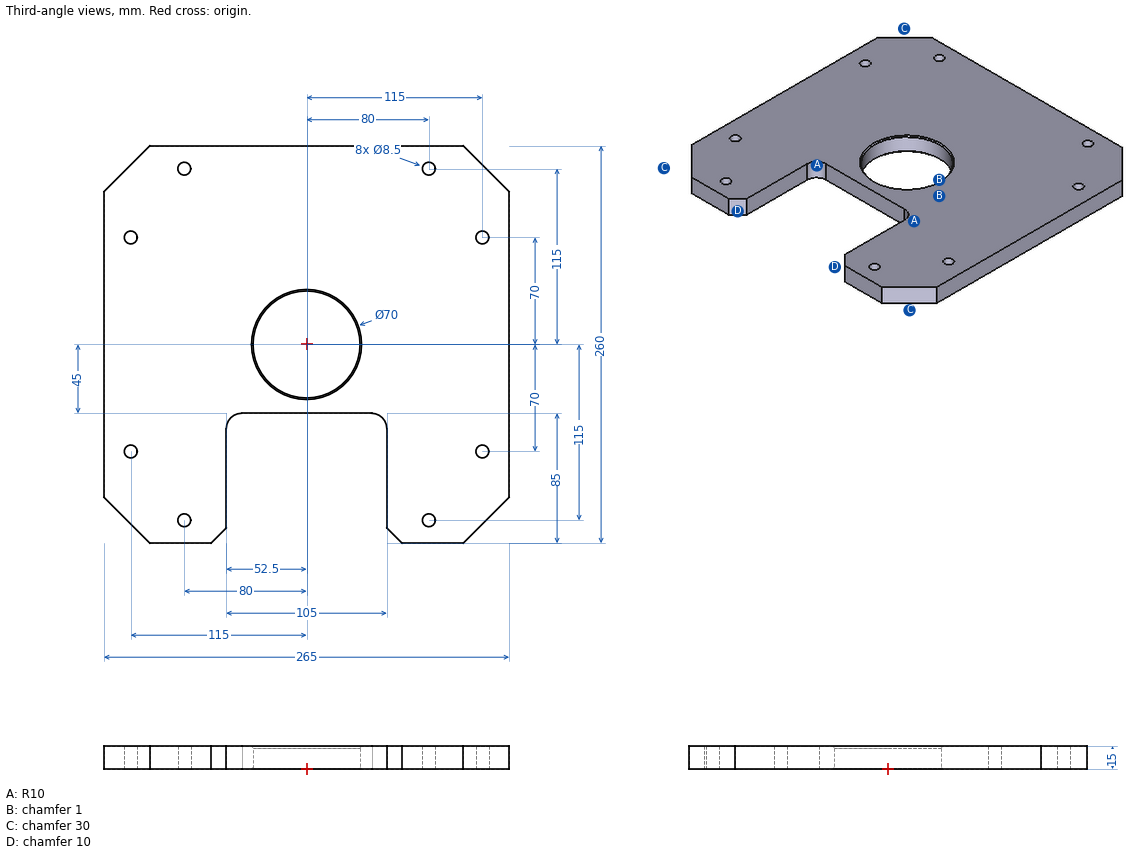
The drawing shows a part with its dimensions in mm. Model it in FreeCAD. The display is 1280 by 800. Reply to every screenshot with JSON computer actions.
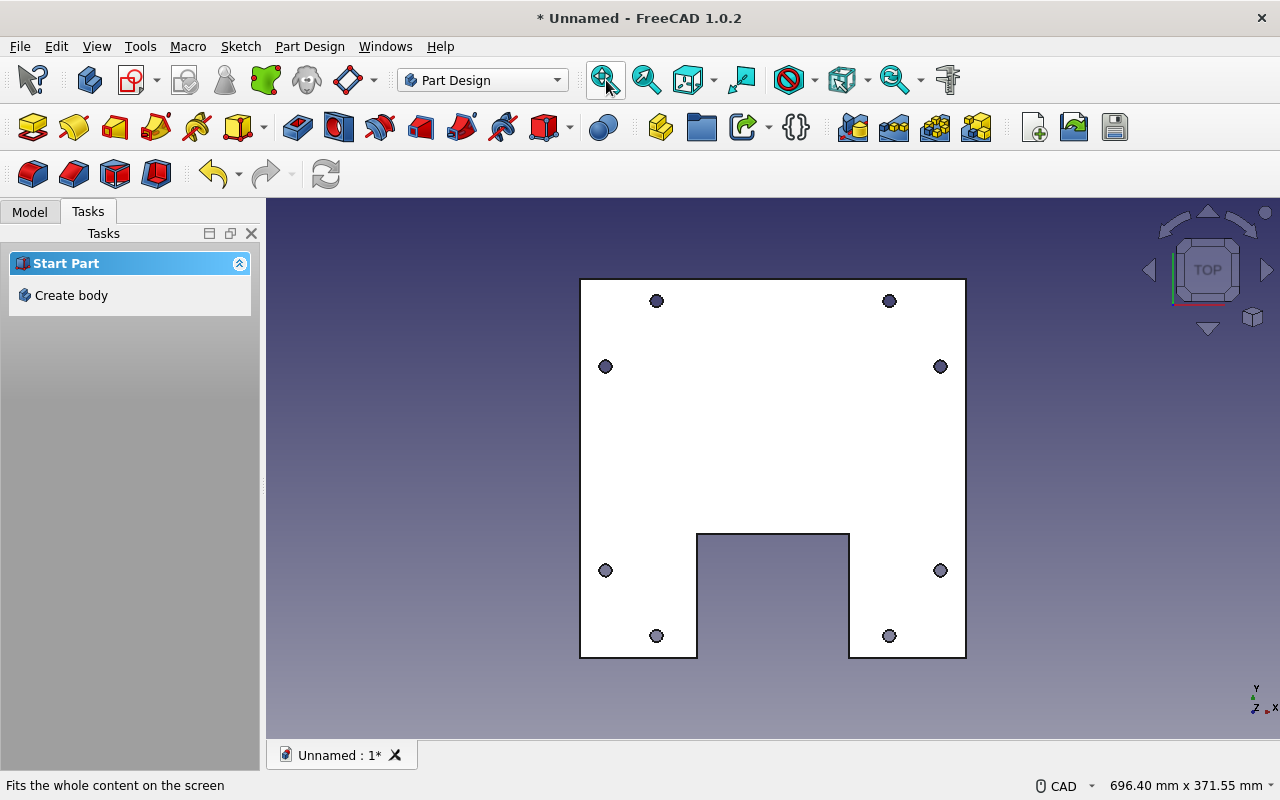
{"action": "scroll", "coordinate": [849, 533], "scroll_direction": "up", "scroll_amount": 4}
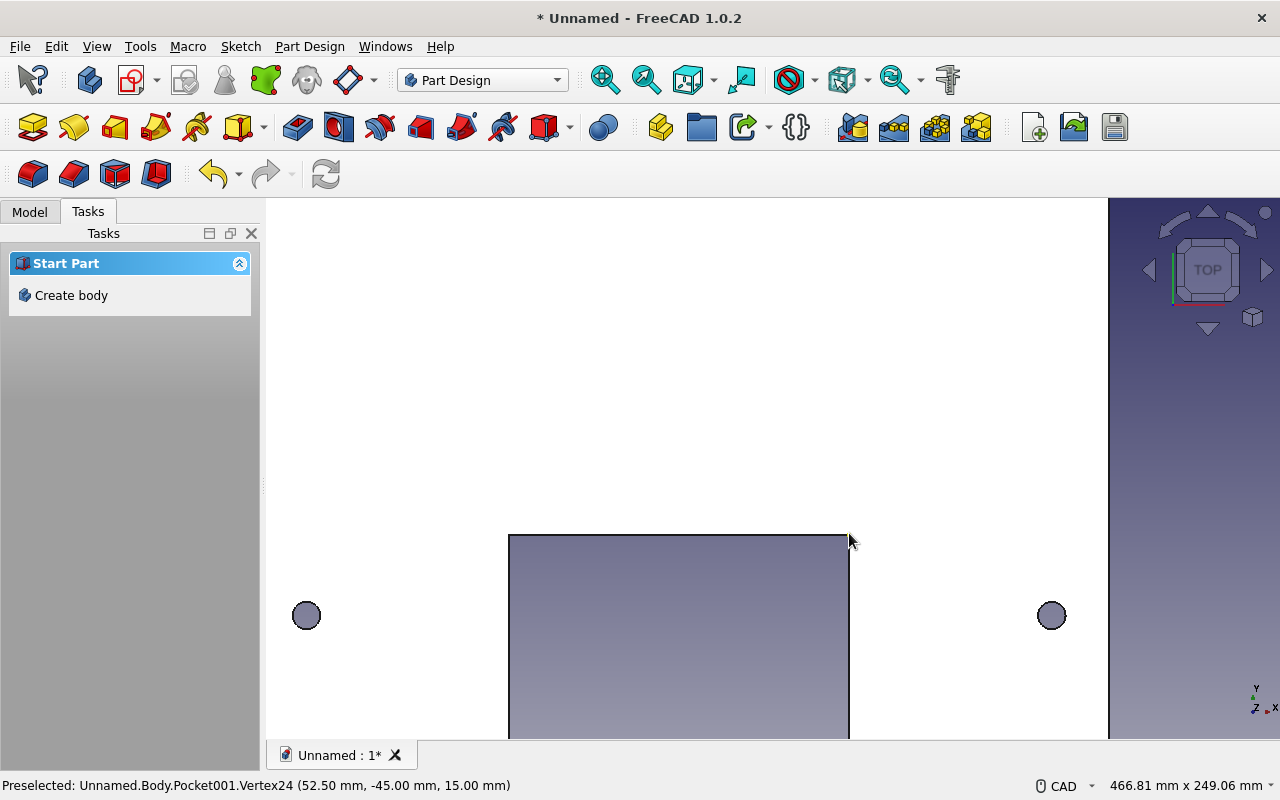
{"action": "left_click", "coordinate": [606, 80]}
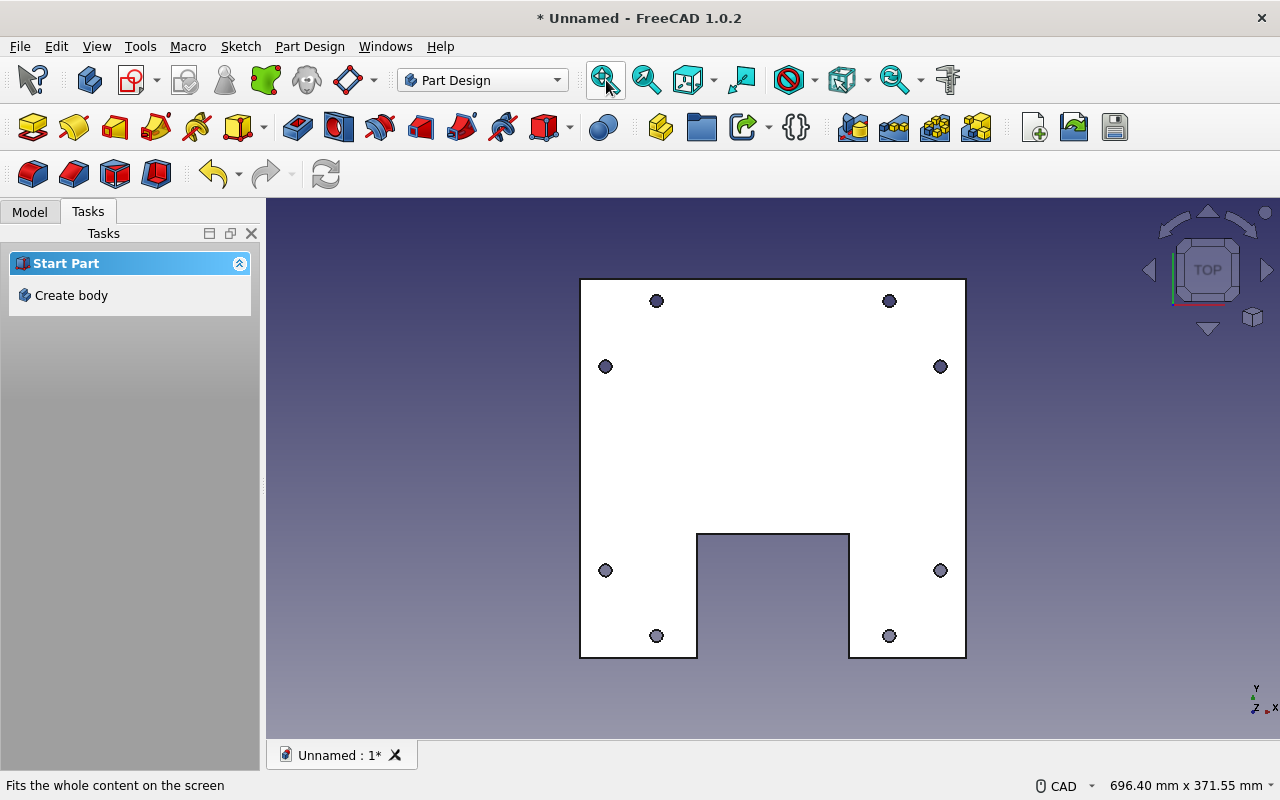
{"action": "key", "text": "1"}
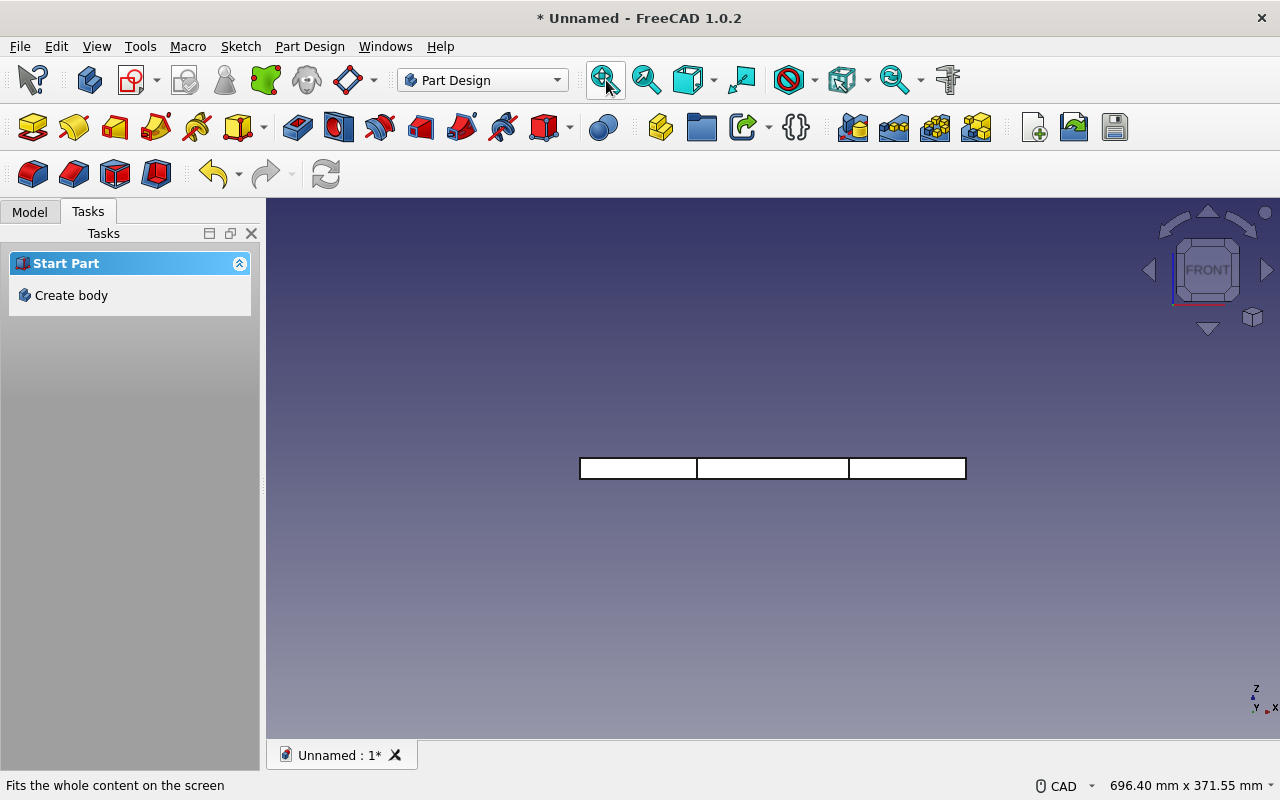
{"action": "key", "text": "v f"}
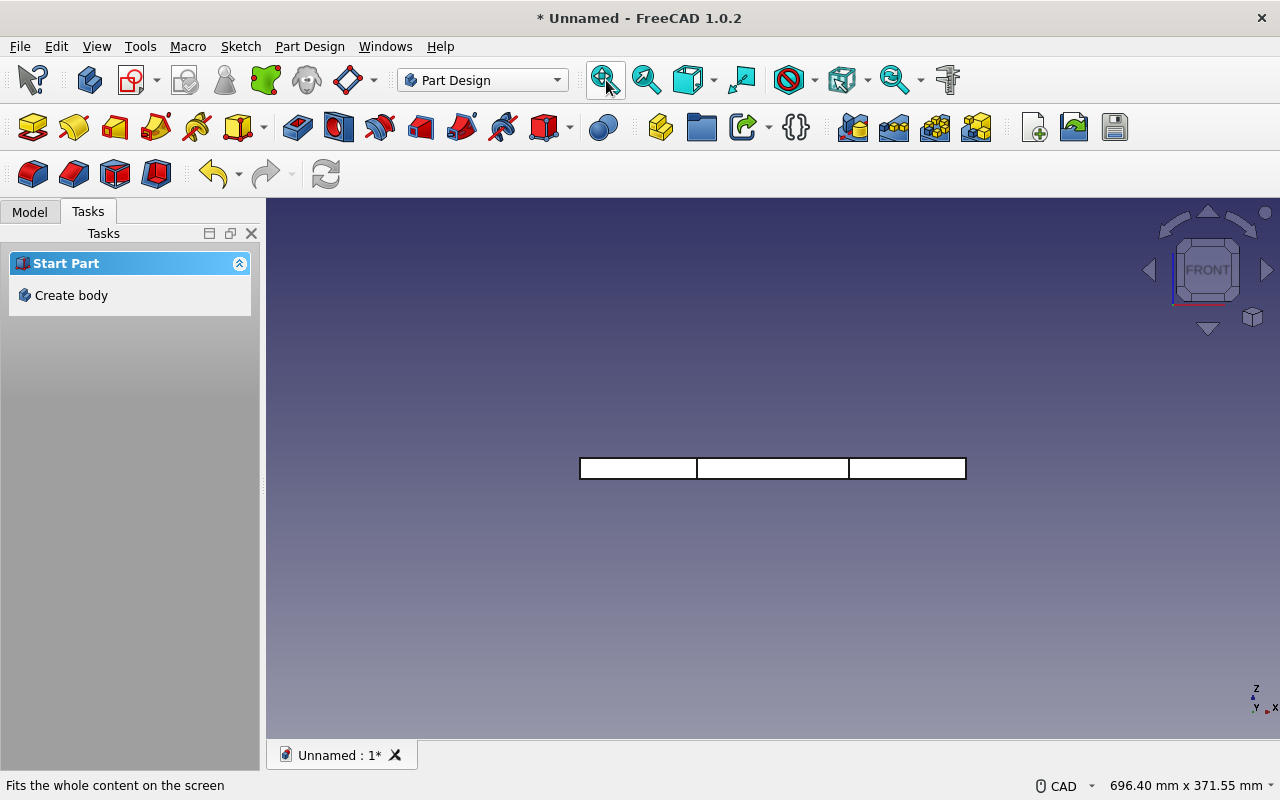
{"action": "scroll", "coordinate": [849, 468], "scroll_direction": "up", "scroll_amount": 4}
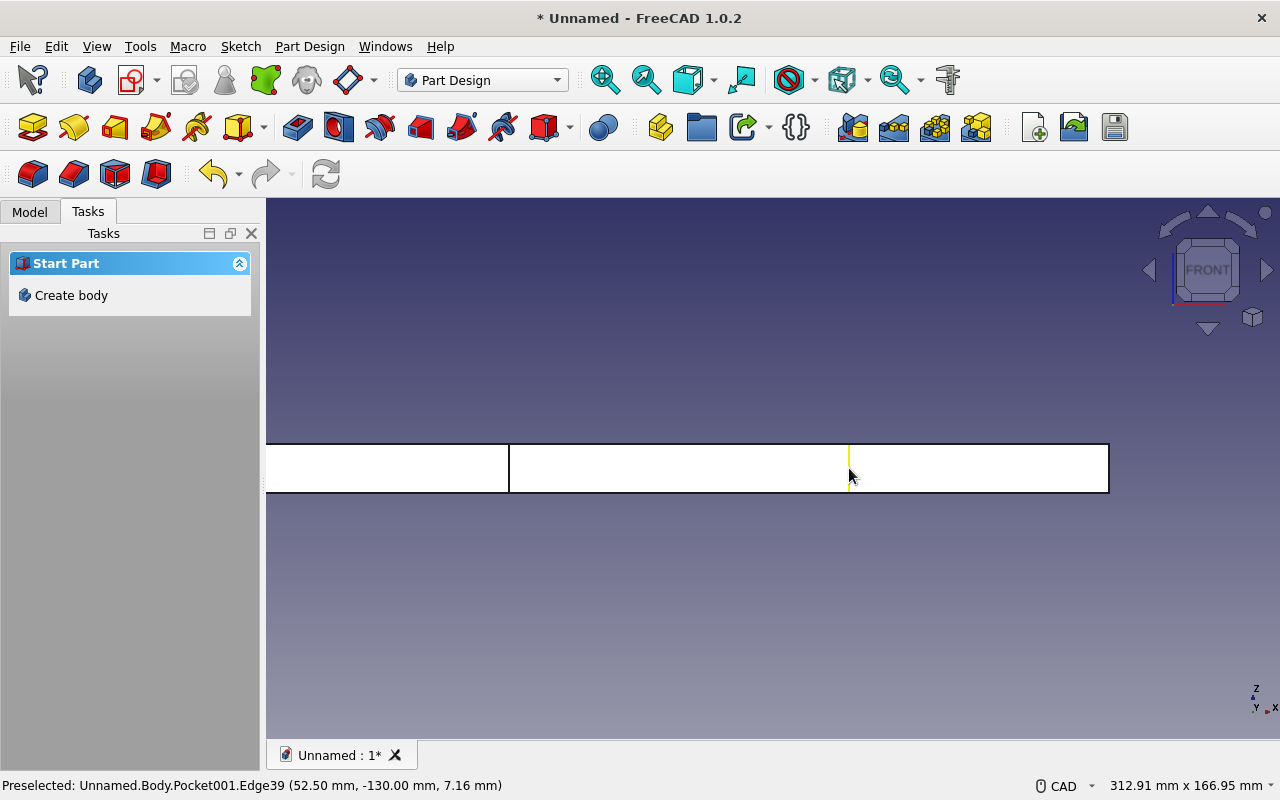
{"action": "left_click", "coordinate": [606, 80]}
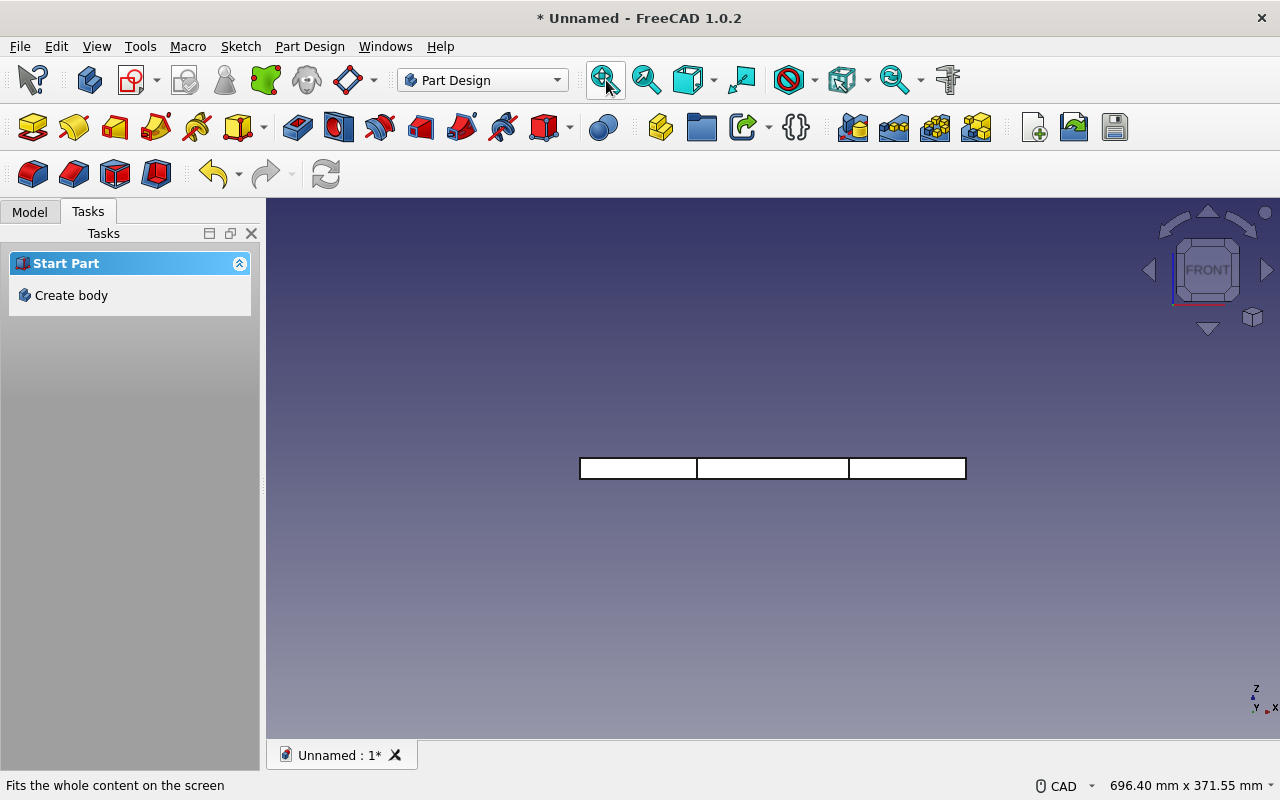
{"action": "key", "text": "3"}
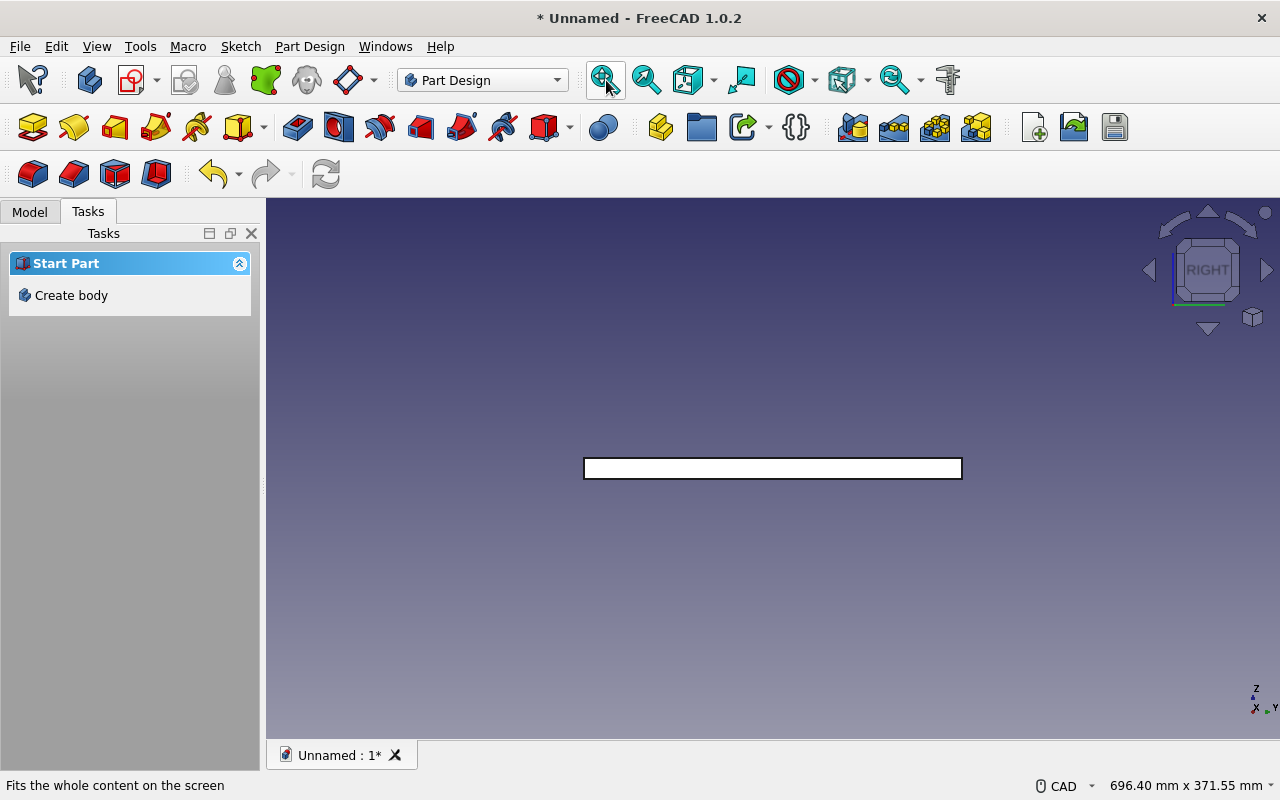
{"action": "key", "text": "v f"}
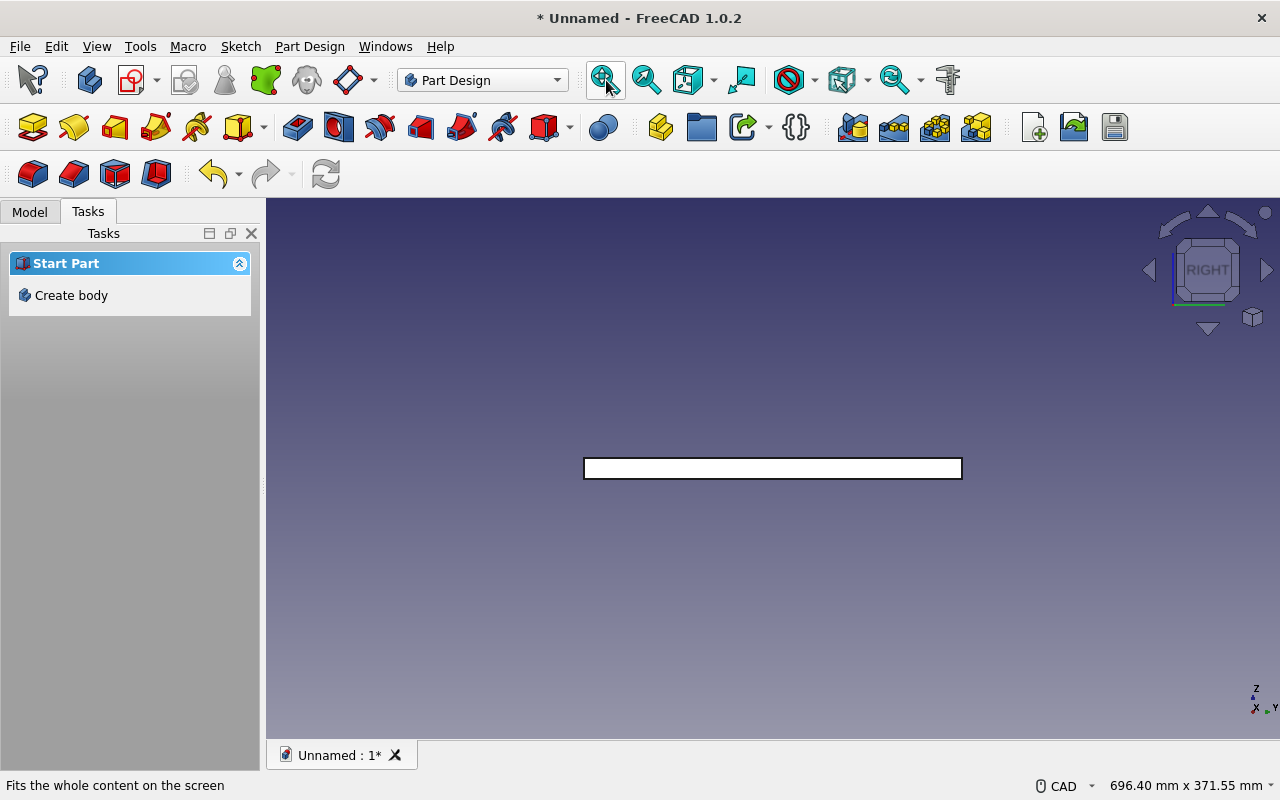
{"action": "scroll", "coordinate": [707, 467], "scroll_direction": "up", "scroll_amount": 4}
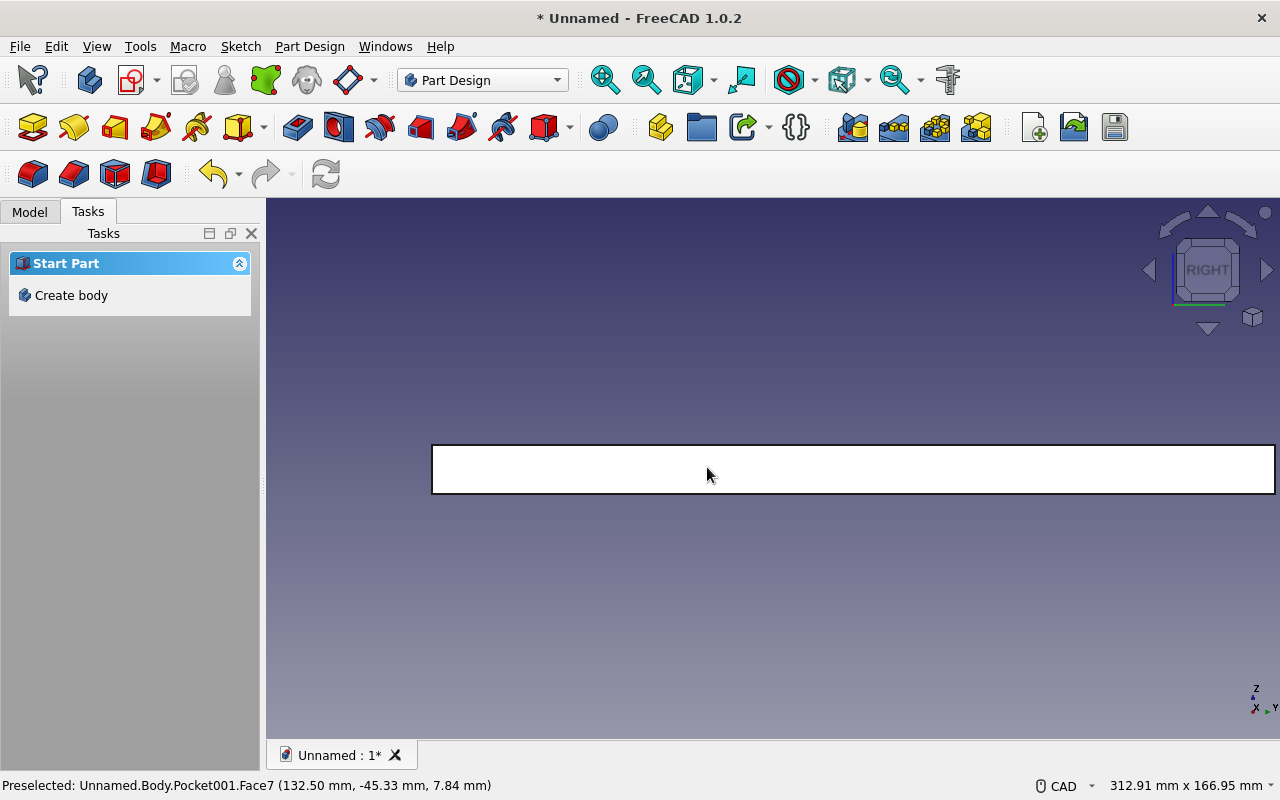
{"action": "key", "text": "v f"}